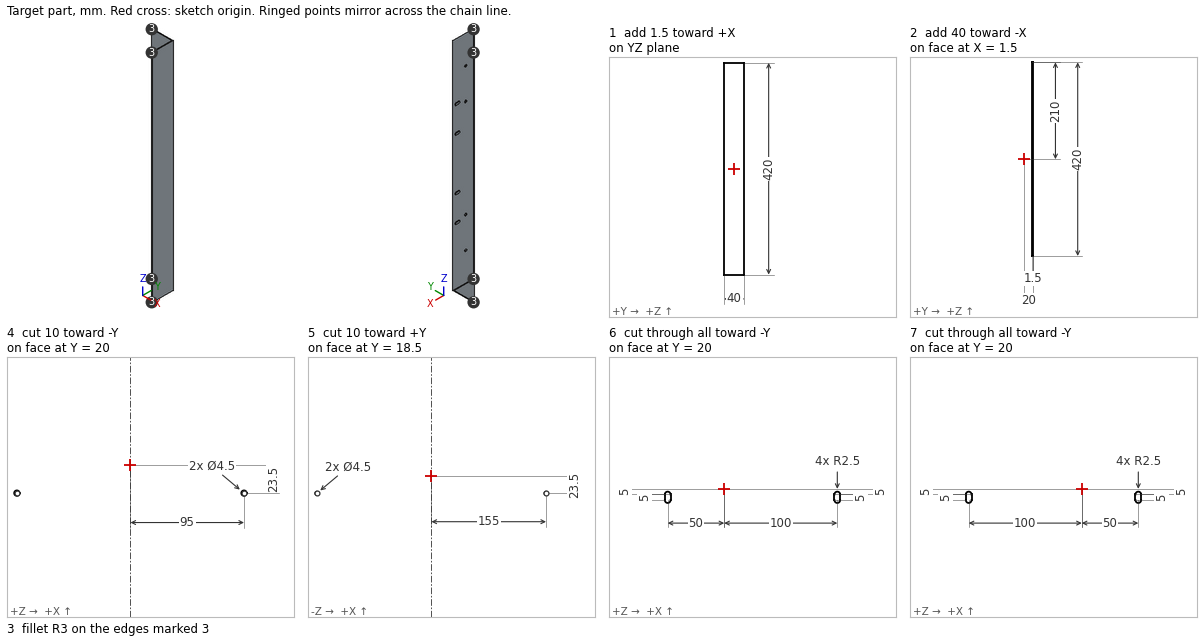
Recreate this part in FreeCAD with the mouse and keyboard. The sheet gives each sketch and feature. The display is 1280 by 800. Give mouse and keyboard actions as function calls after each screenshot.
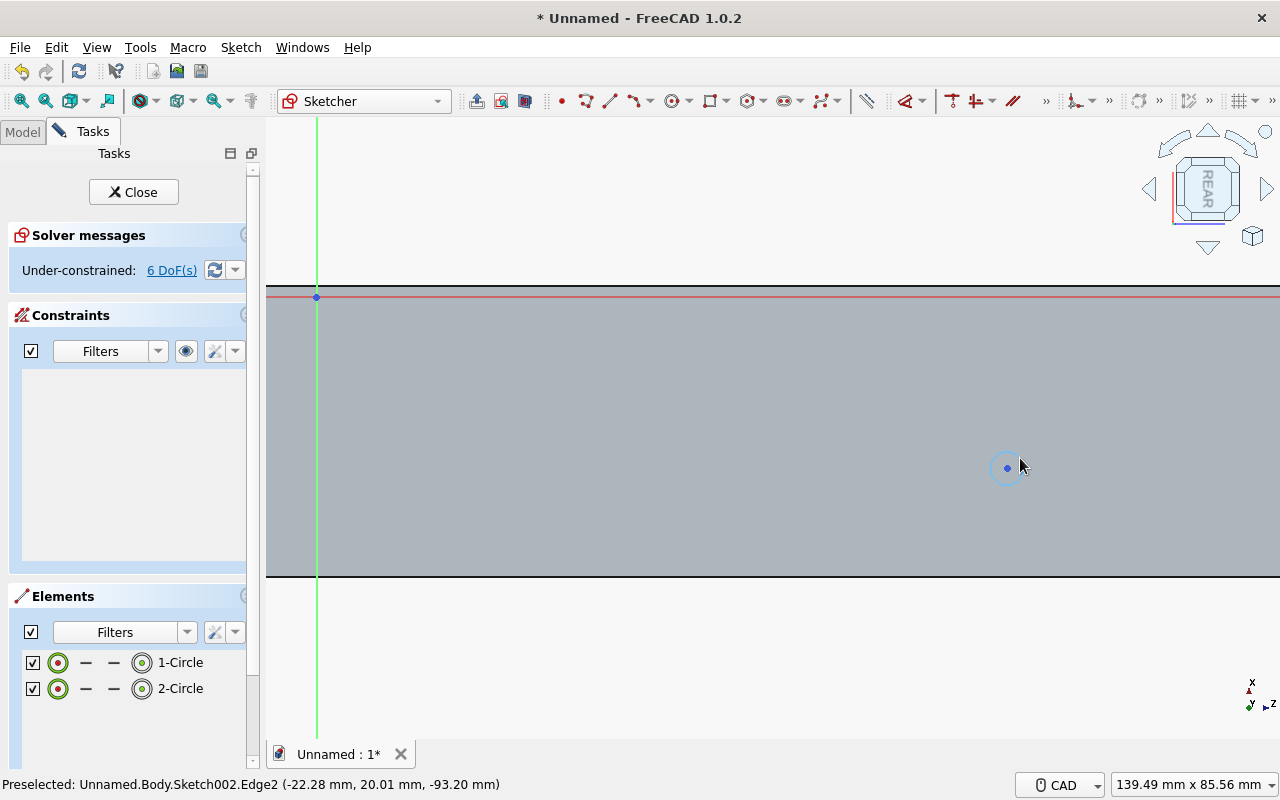
click(1019, 457)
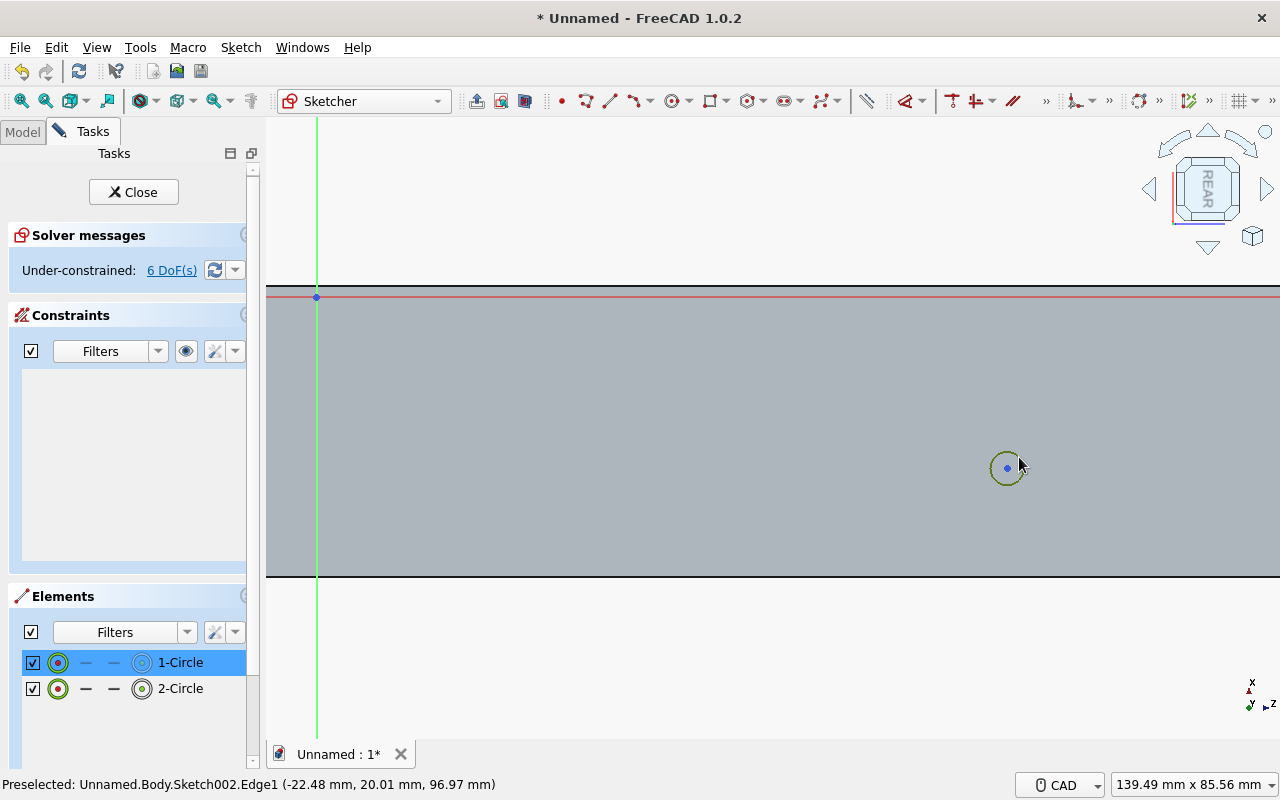
scroll(1021, 458, down, 4)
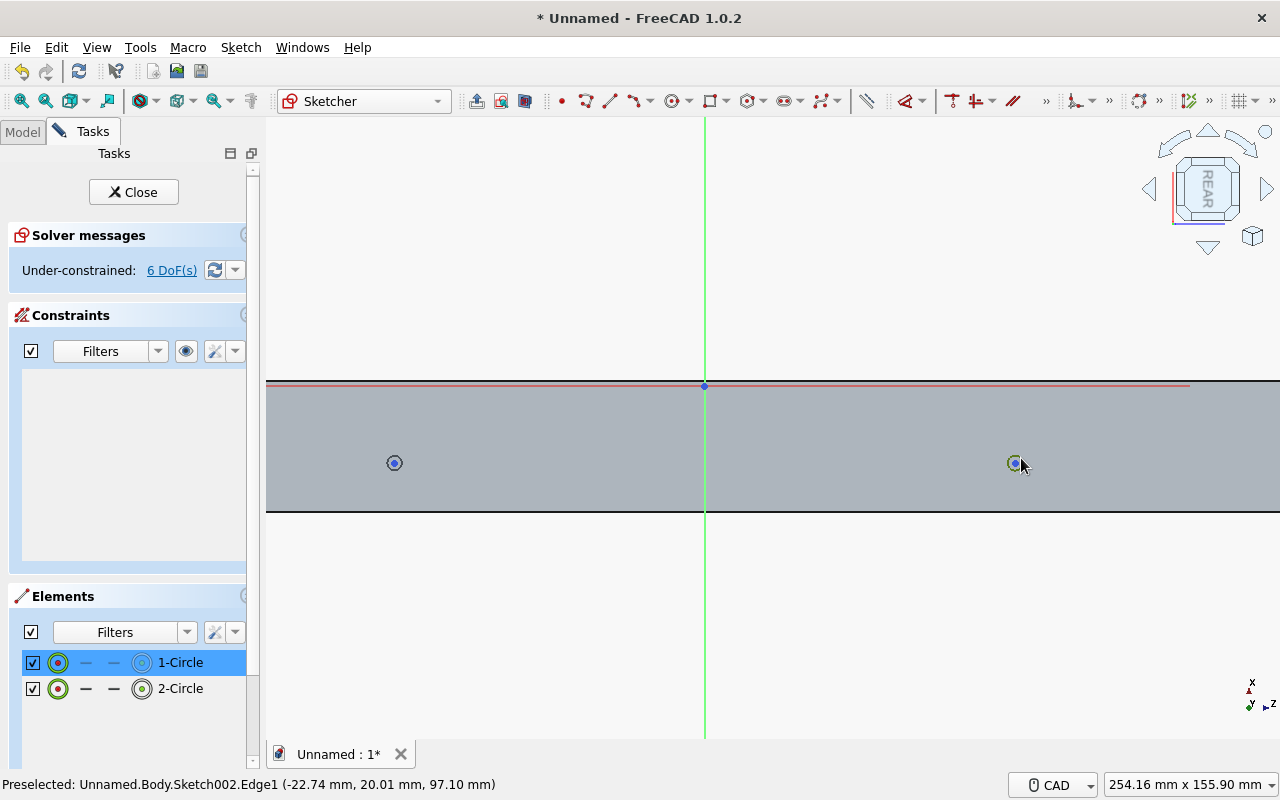
scroll(400, 458, up, 4)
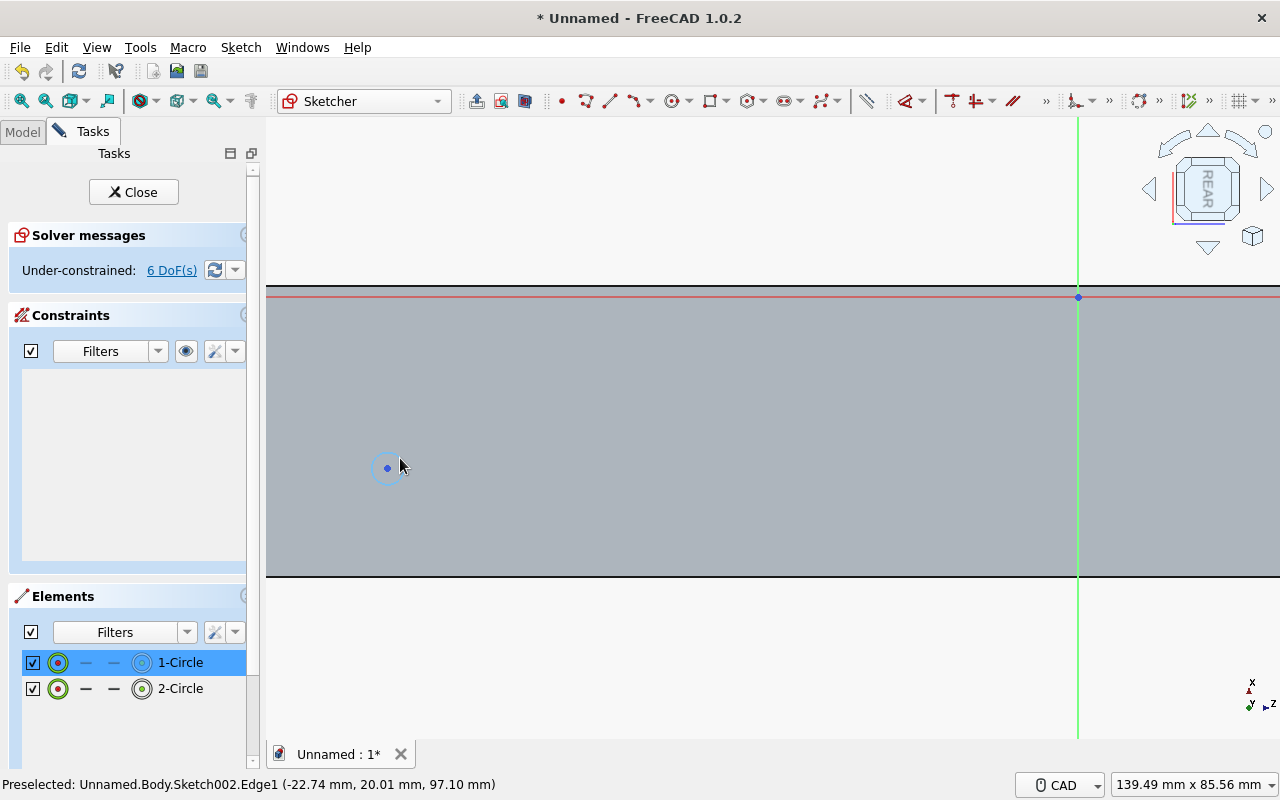
click(399, 457)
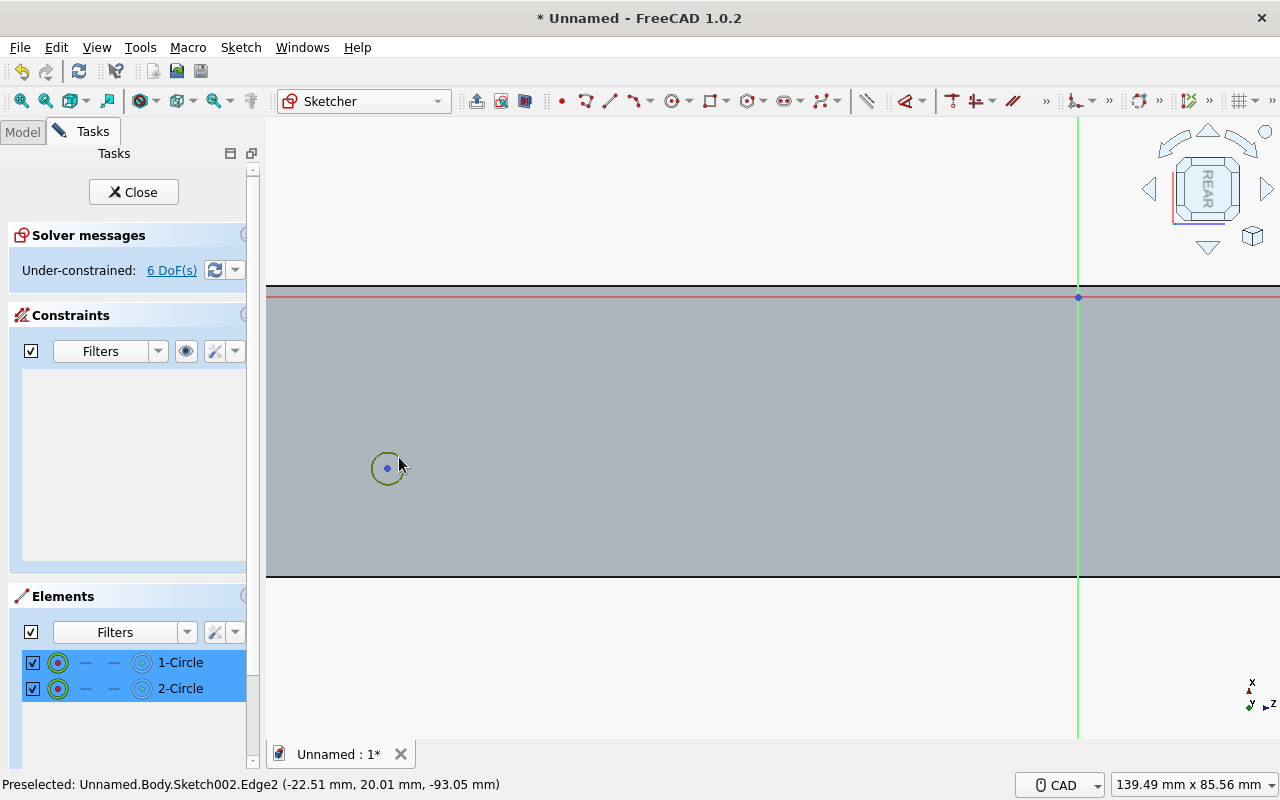
key(e)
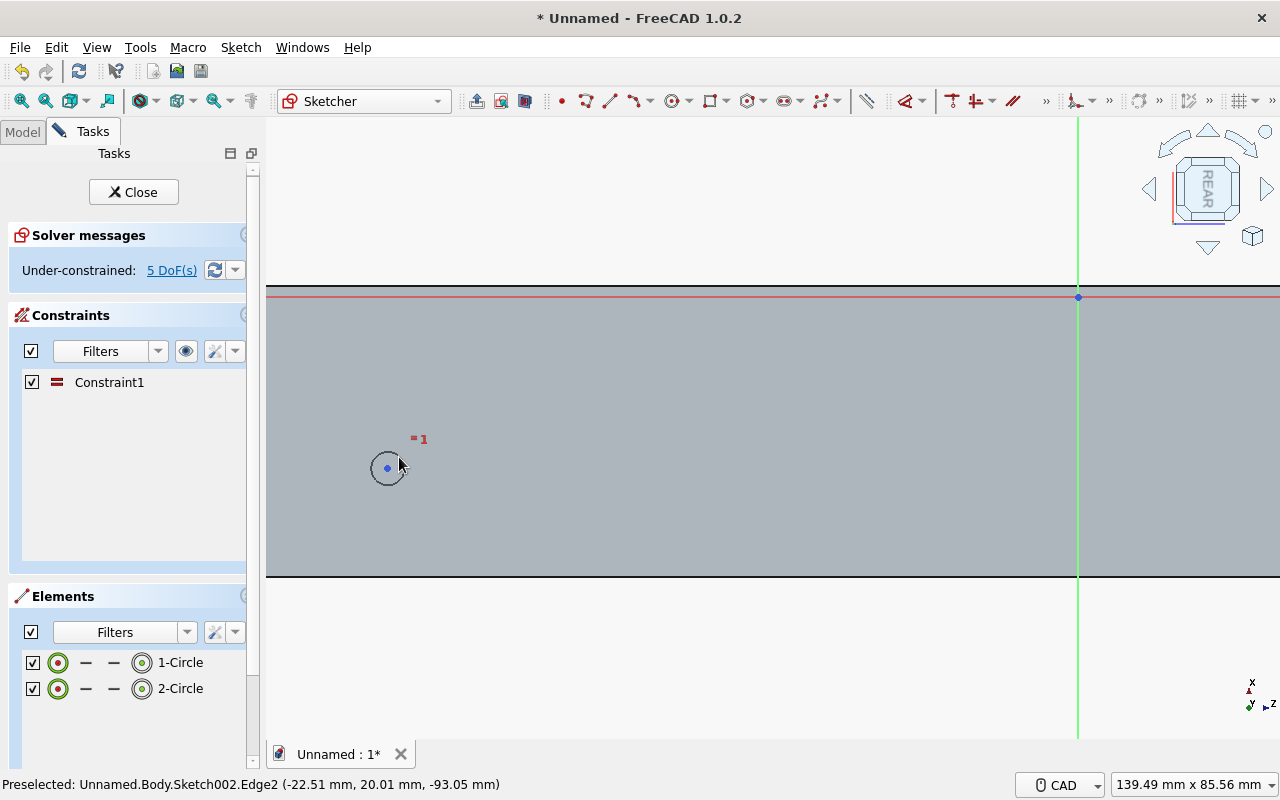
scroll(399, 458, down, 4)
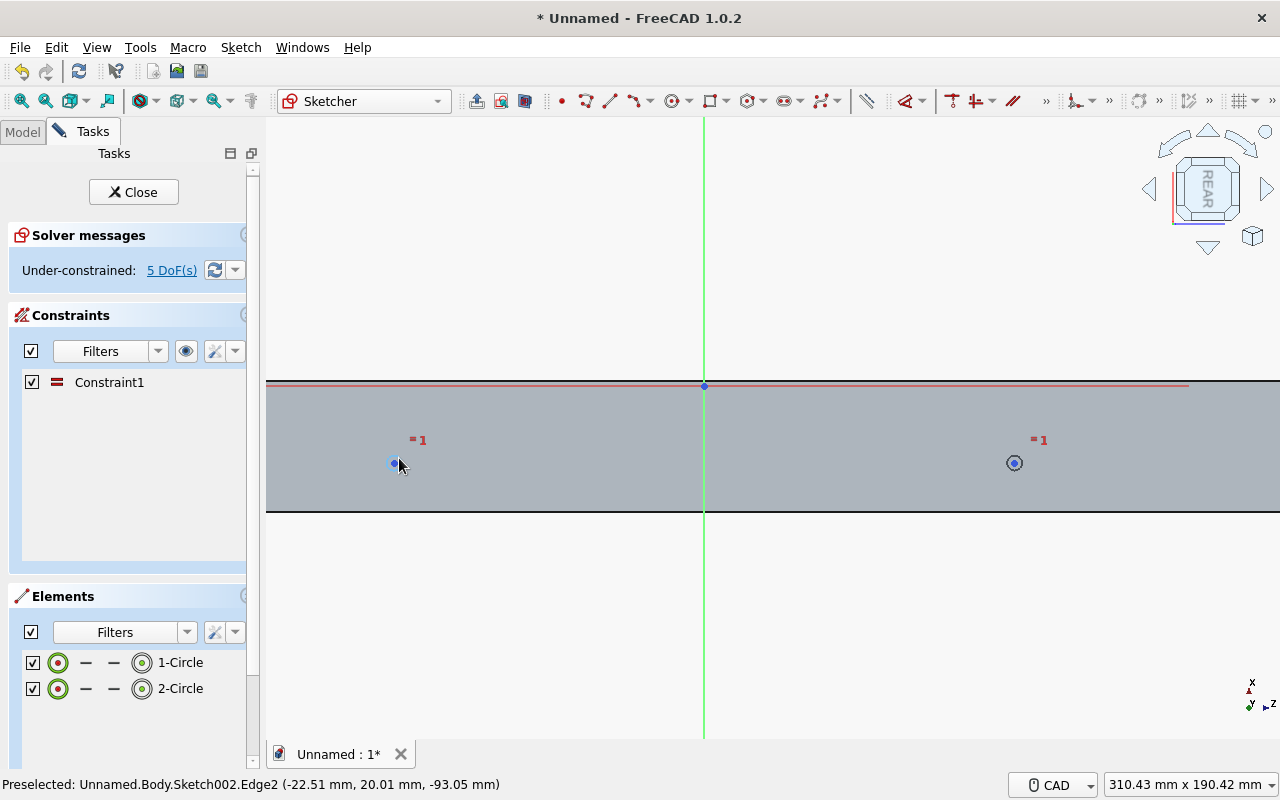
click(1015, 463)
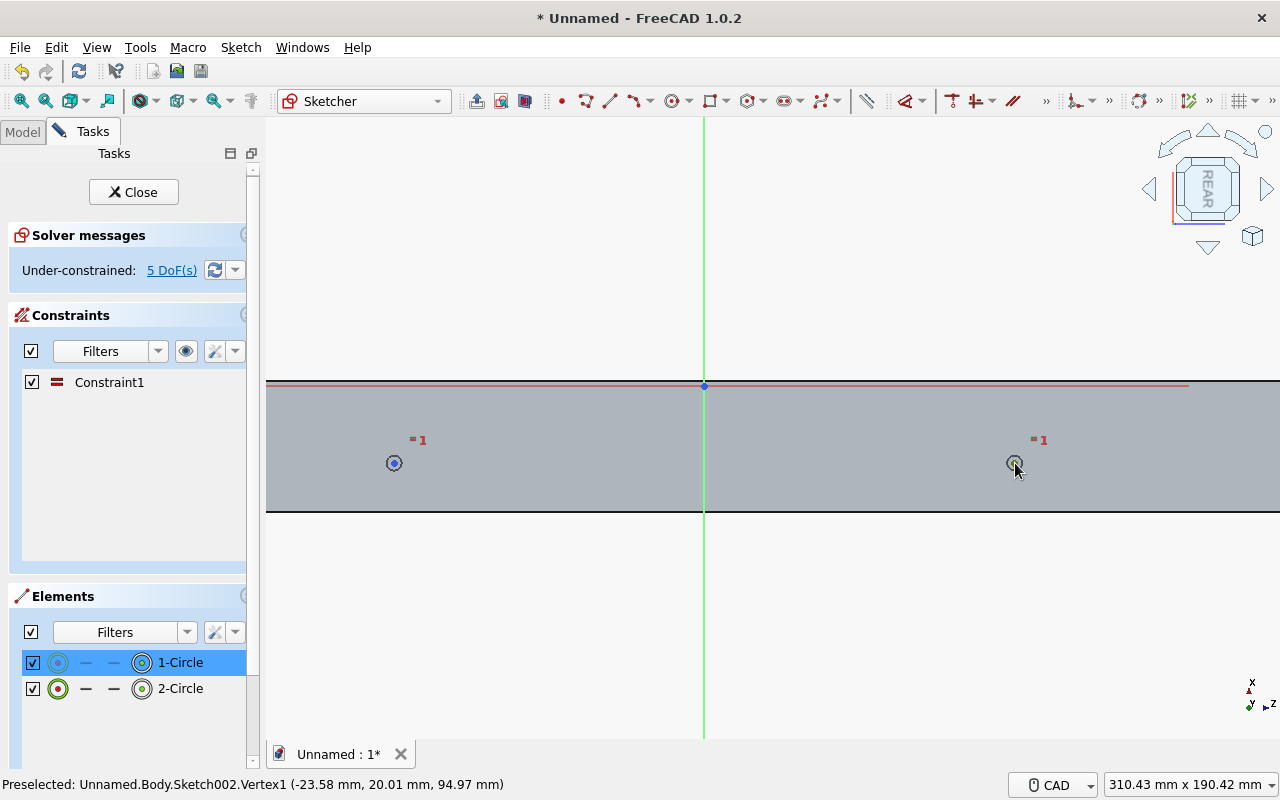
click(394, 463)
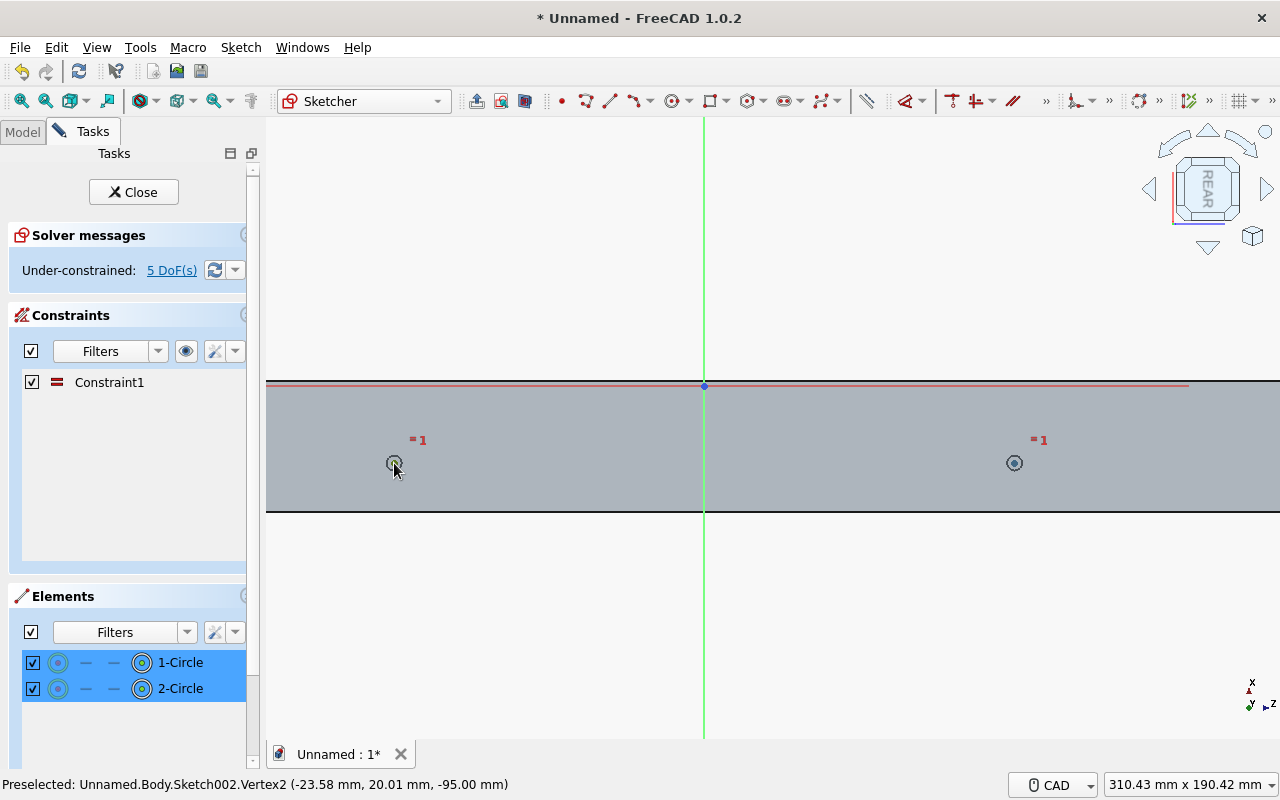
click(704, 671)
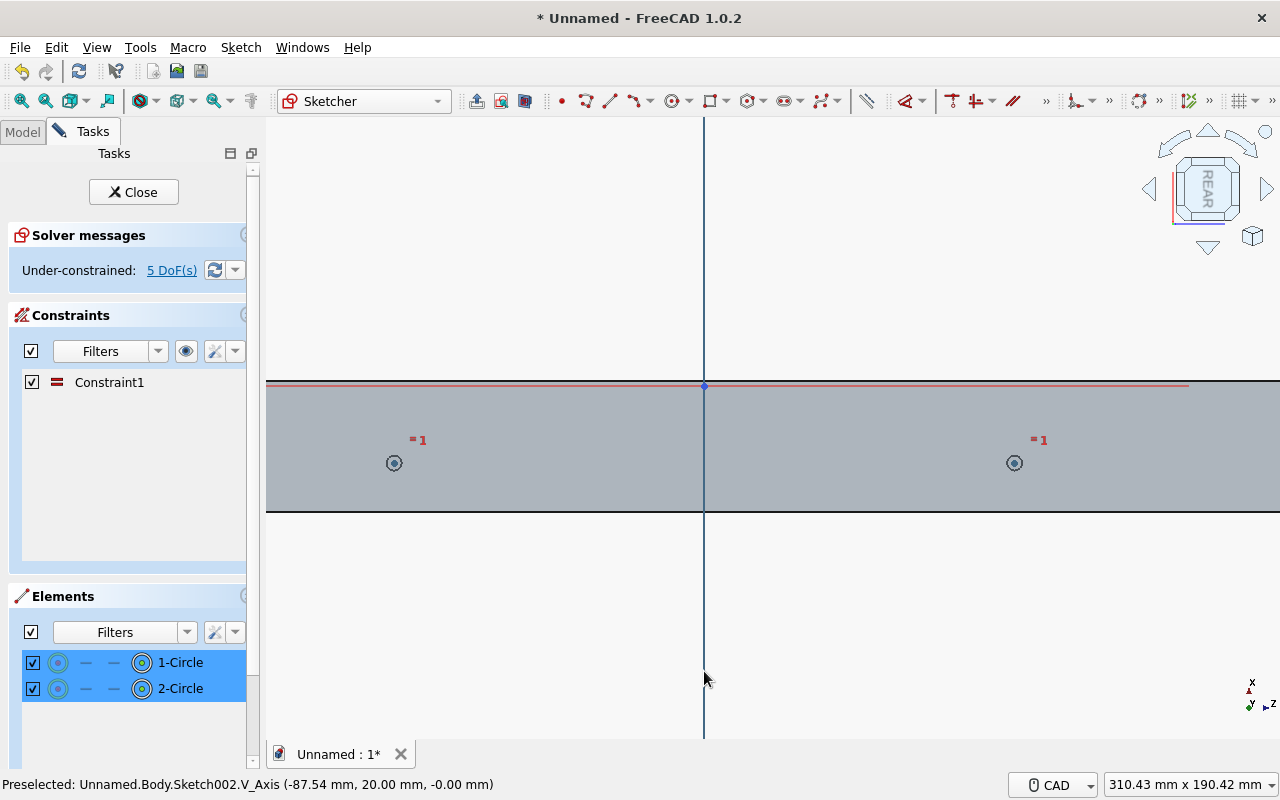
key(s)